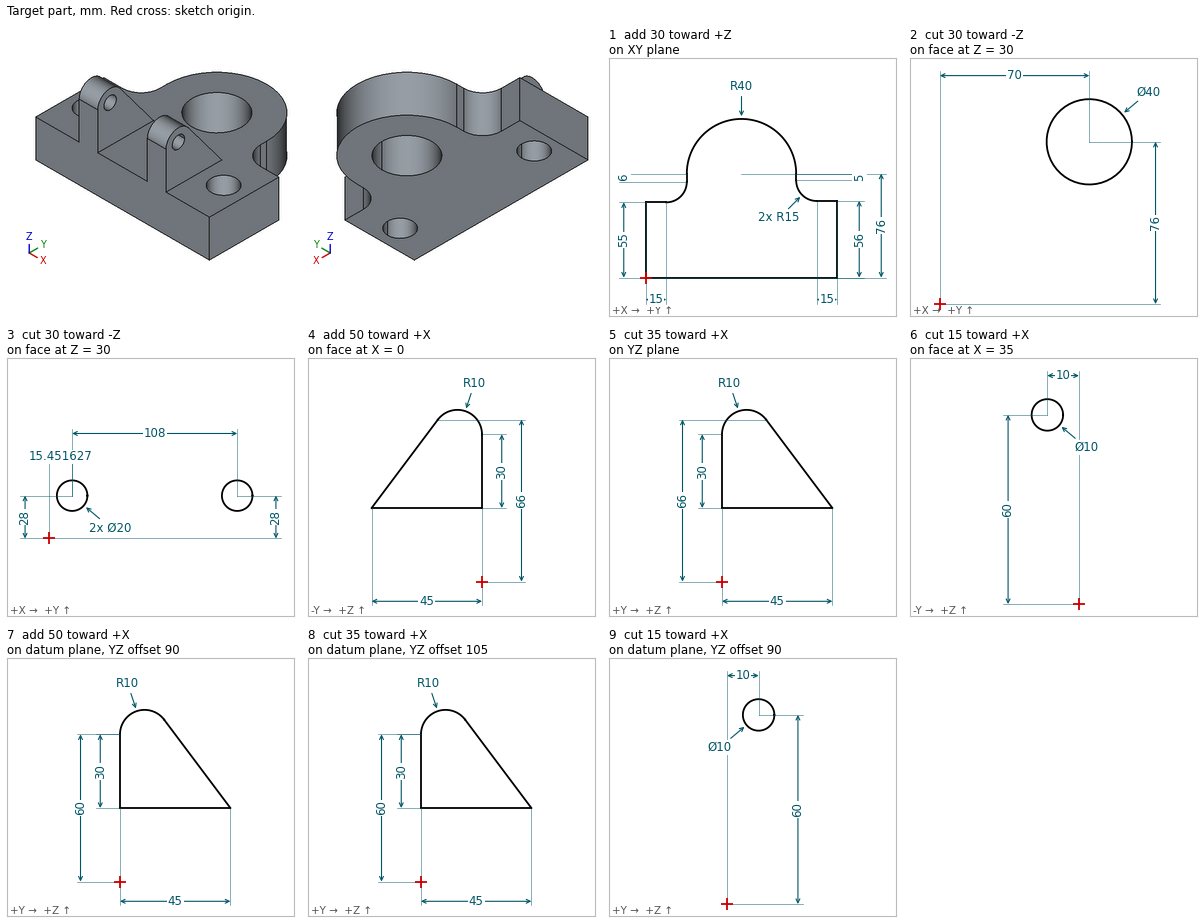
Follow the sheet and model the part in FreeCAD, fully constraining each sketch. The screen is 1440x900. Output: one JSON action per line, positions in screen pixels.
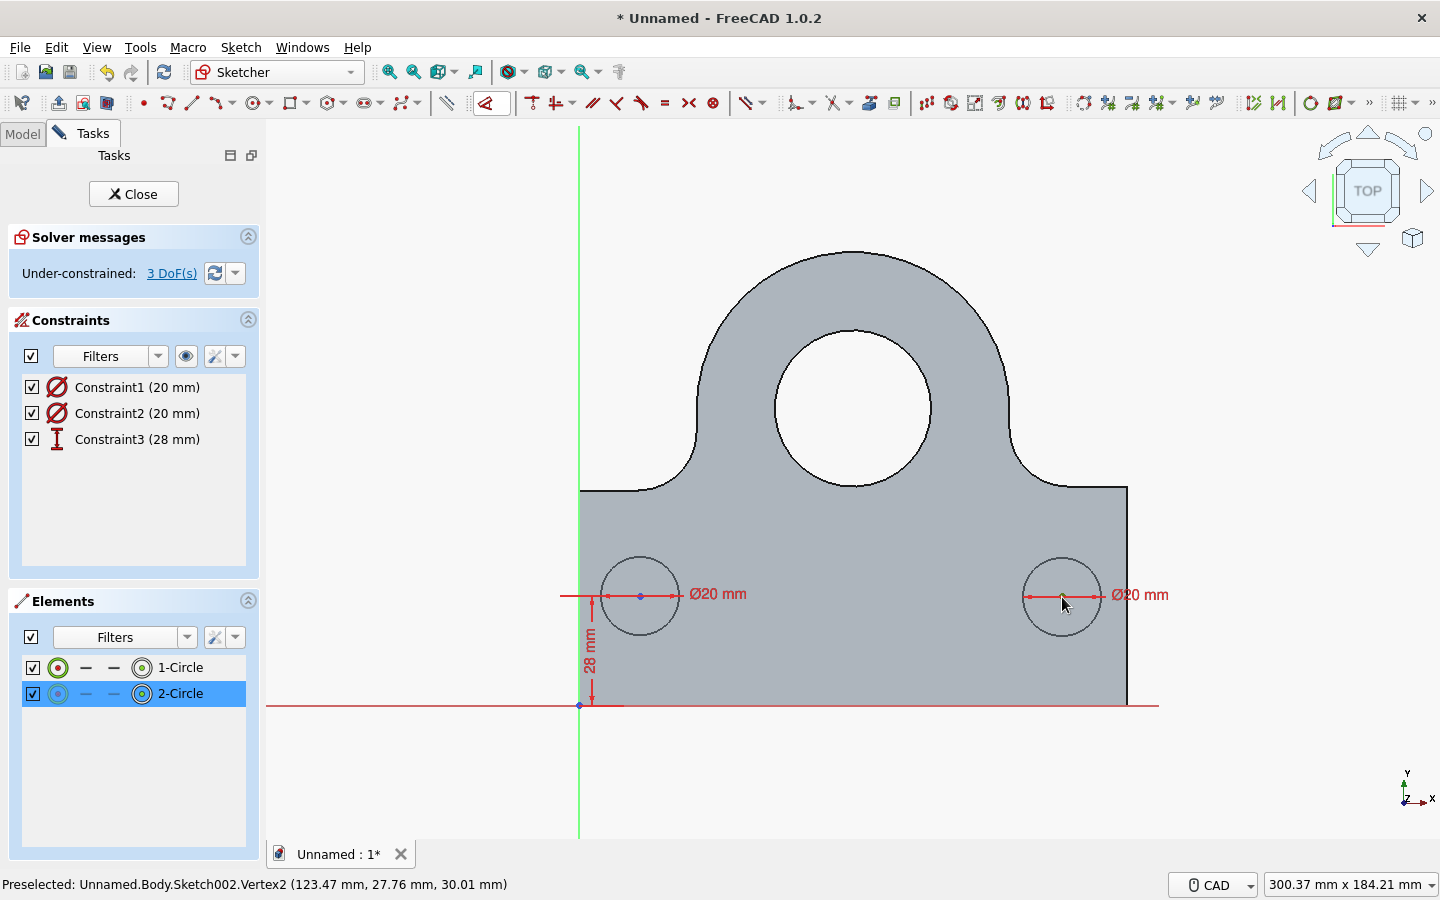
{"action": "key", "text": "i"}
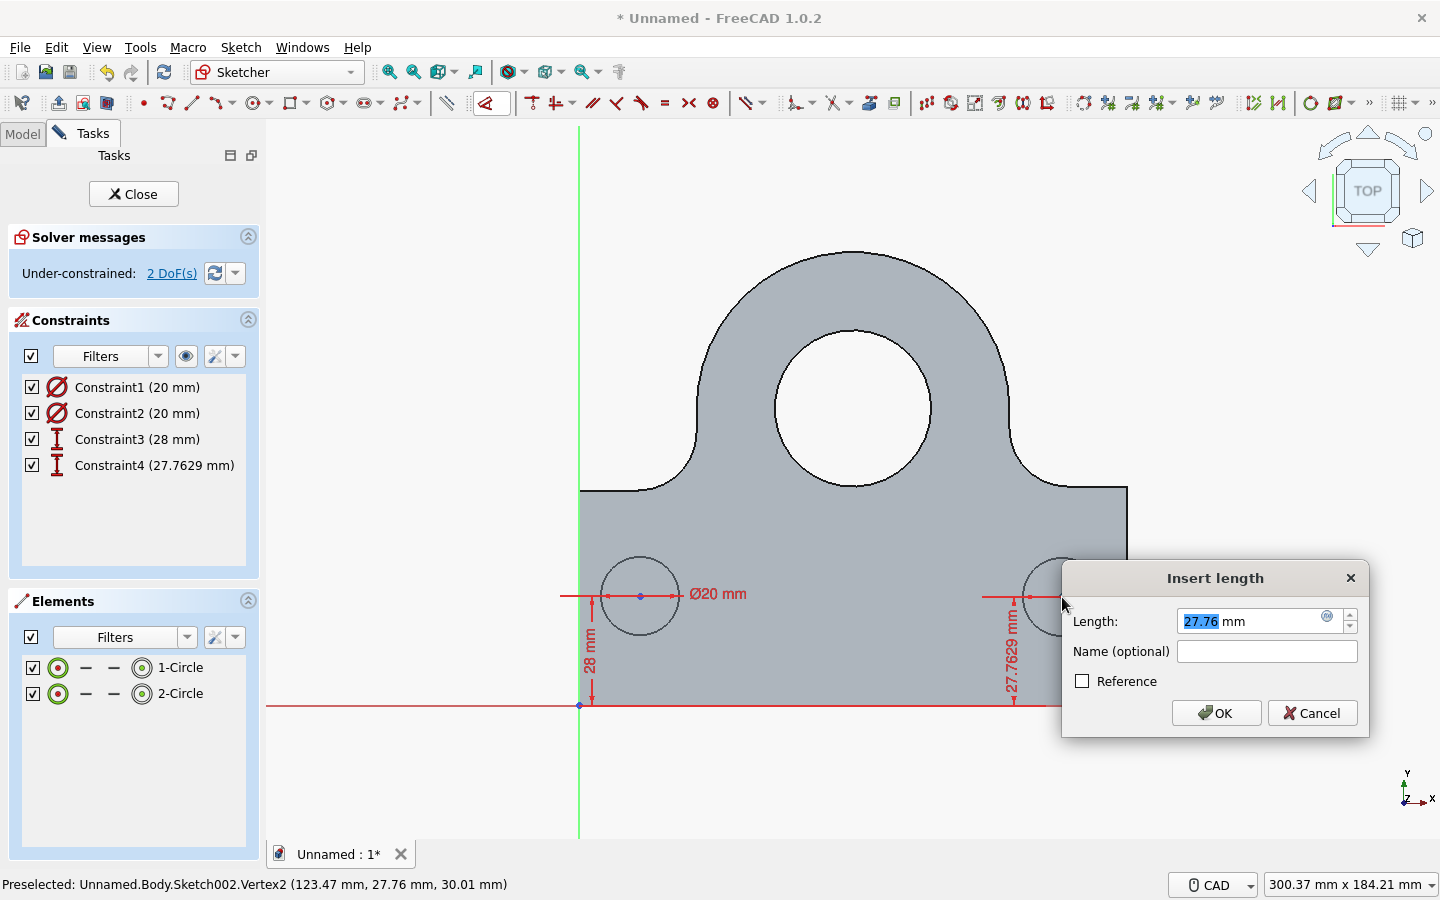
{"action": "type", "text": "28"}
{"action": "key", "text": "Return"}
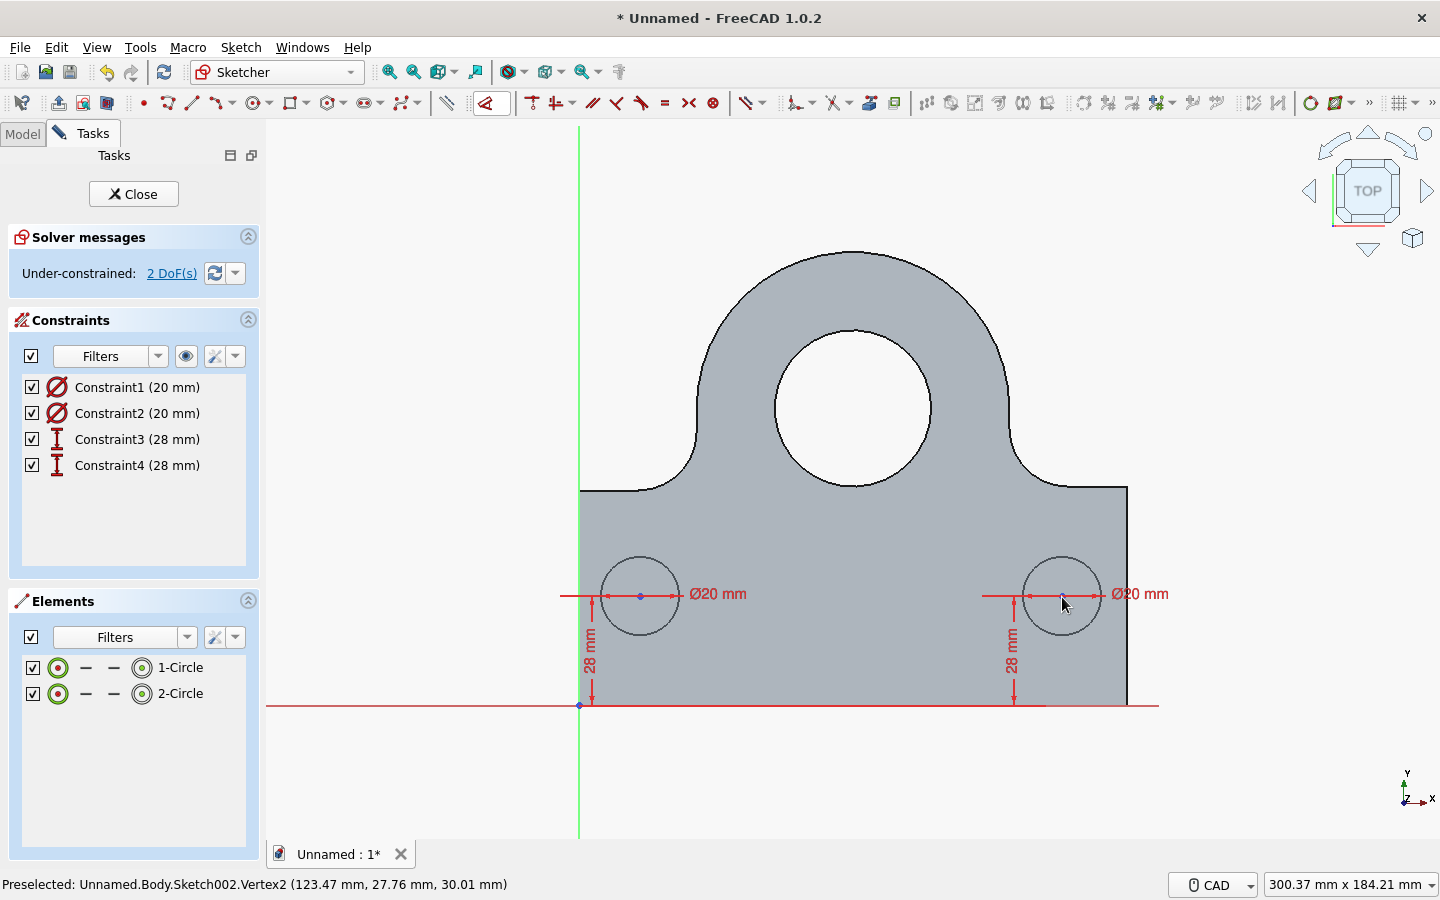
{"action": "left_click", "coordinate": [640, 596]}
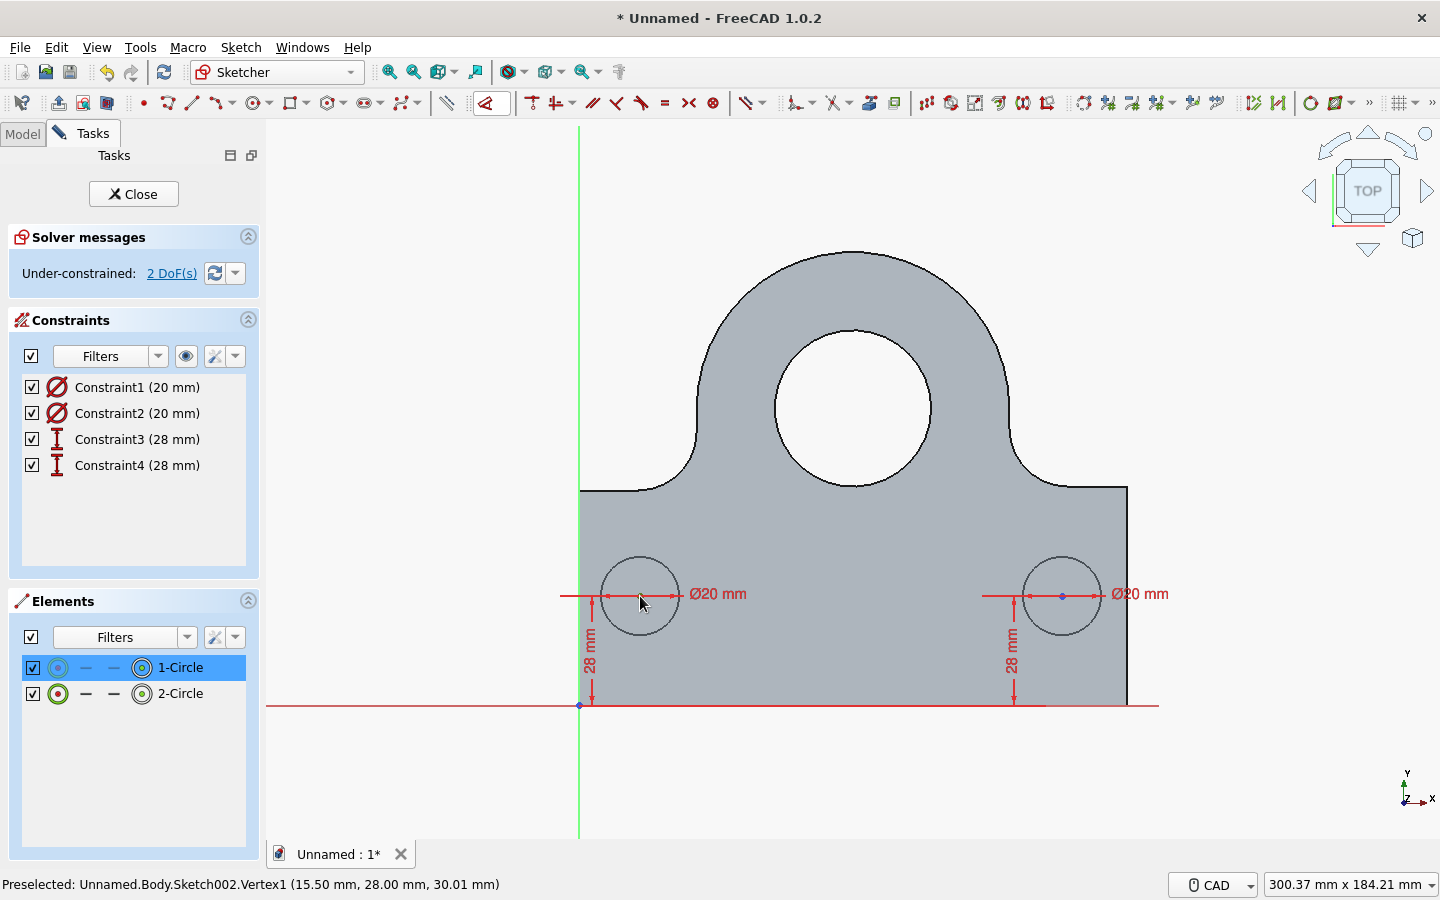
{"action": "left_click", "coordinate": [1062, 596]}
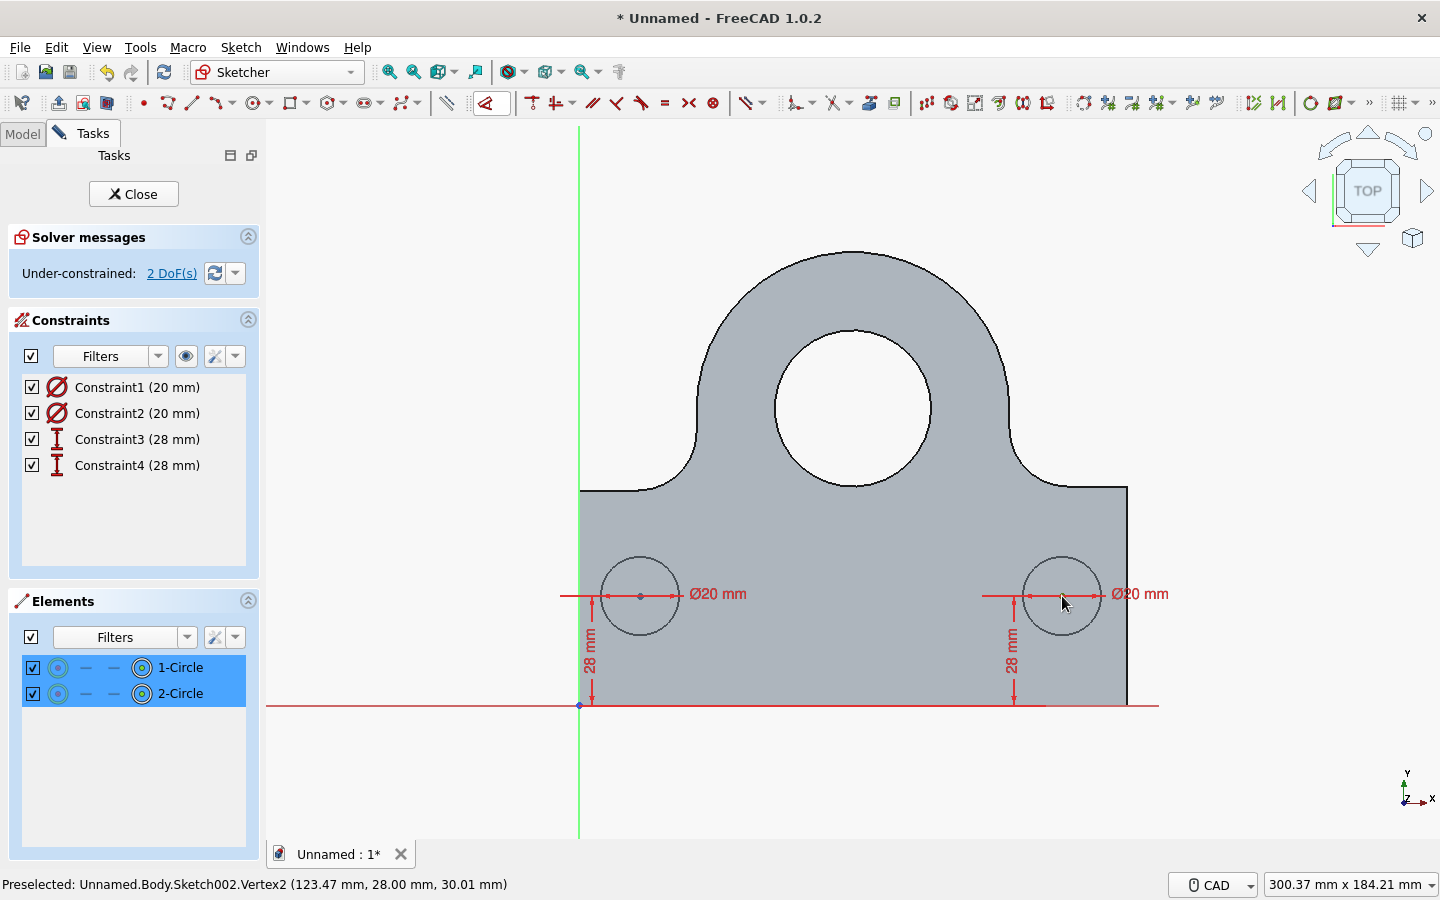
{"action": "key", "text": "l"}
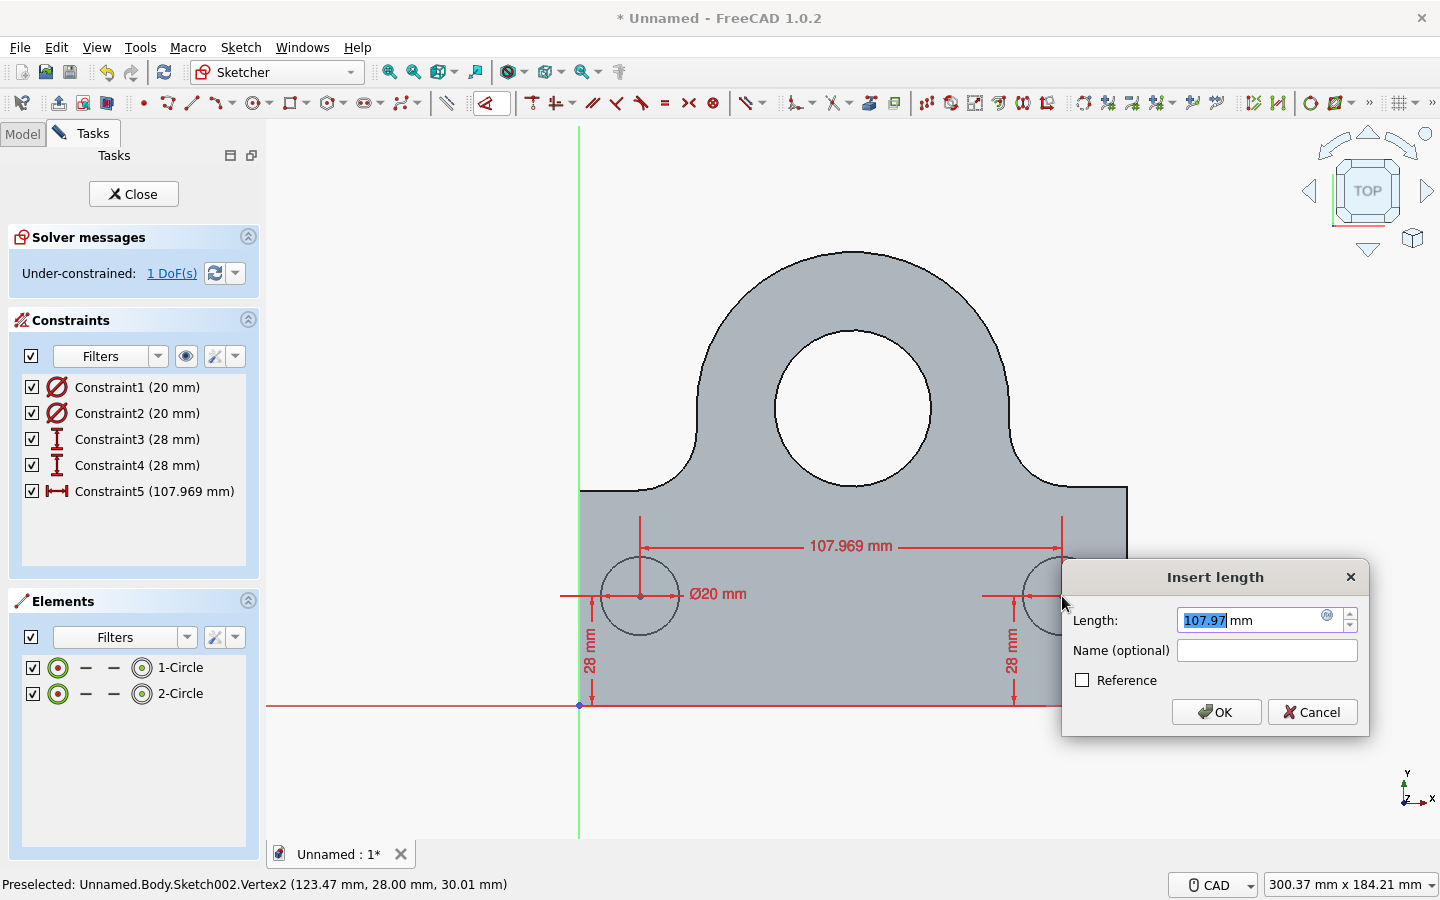
{"action": "type", "text": "108"}
{"action": "key", "text": "Return"}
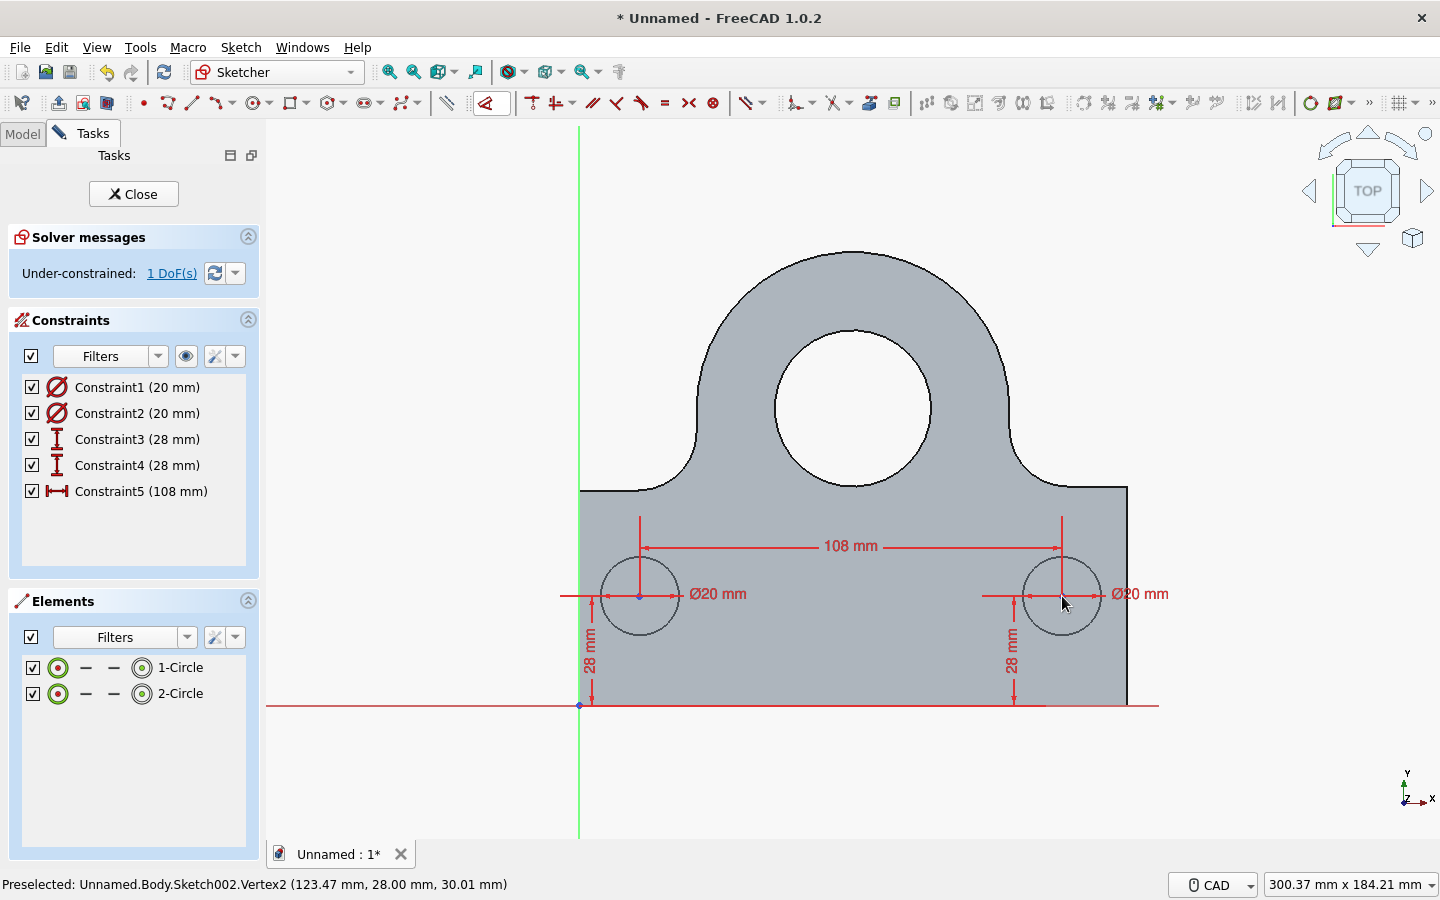
{"action": "left_click", "coordinate": [640, 596]}